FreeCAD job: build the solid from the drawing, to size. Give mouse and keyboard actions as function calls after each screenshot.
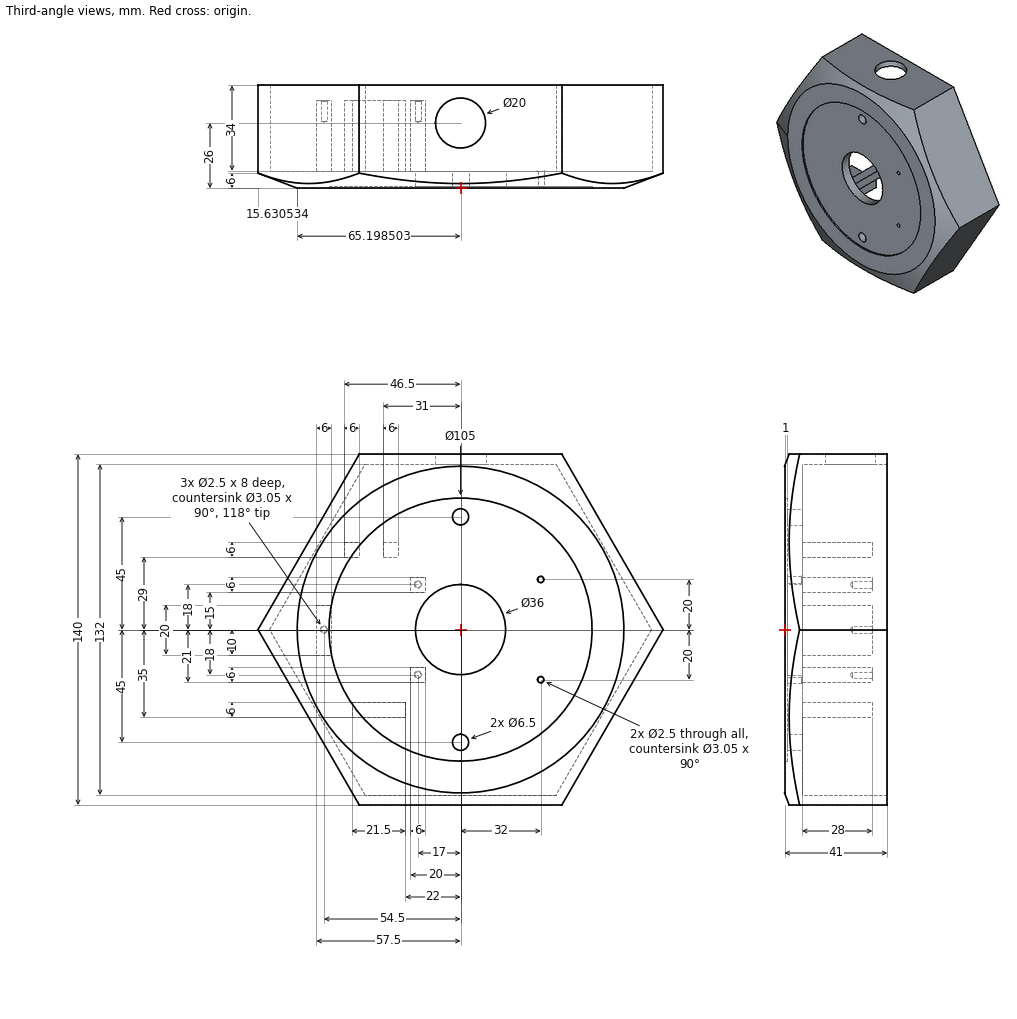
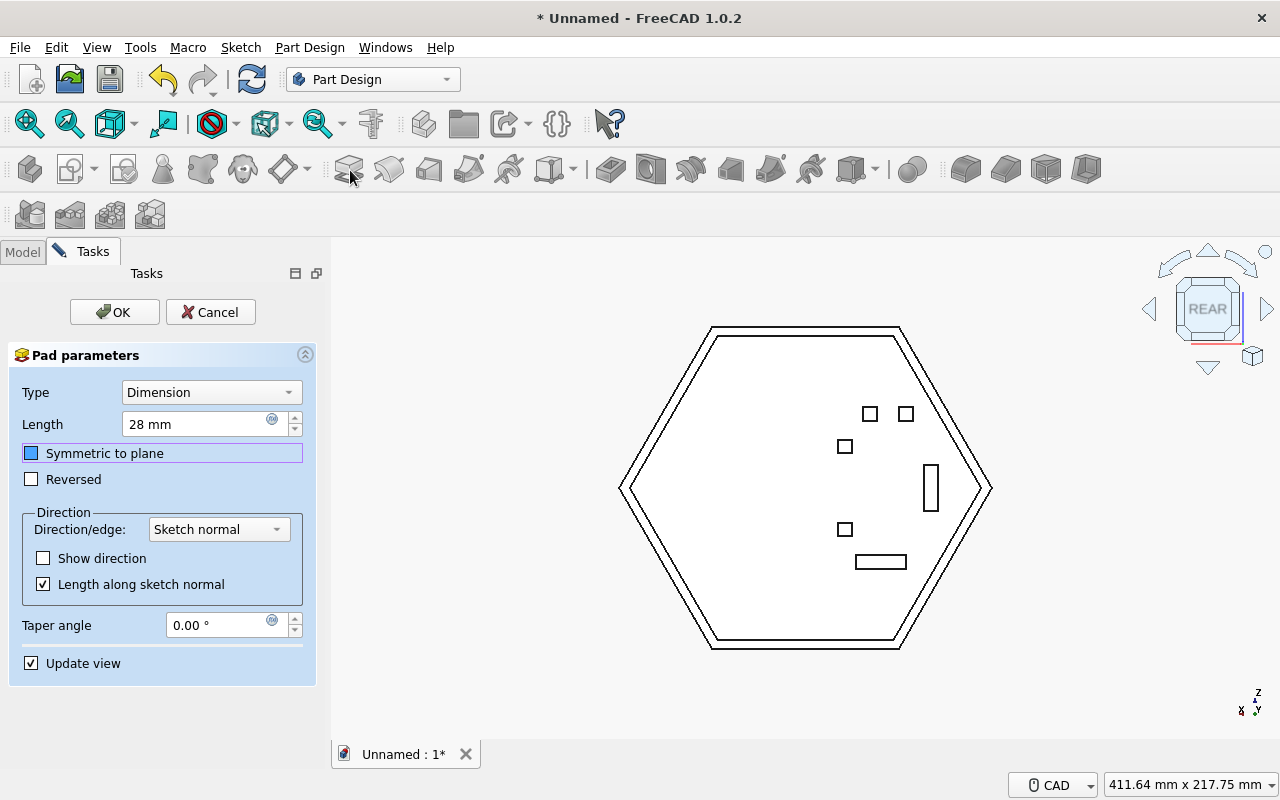
click(115, 312)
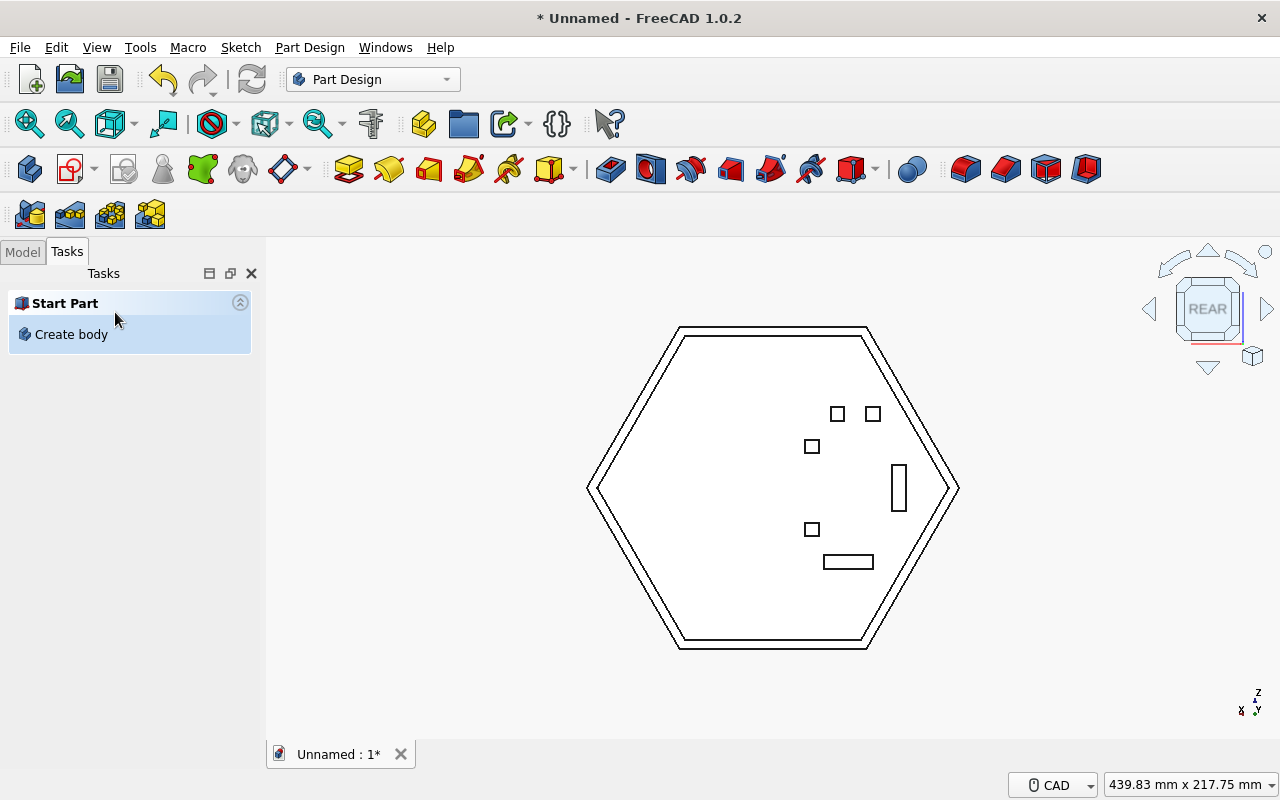
click(723, 487)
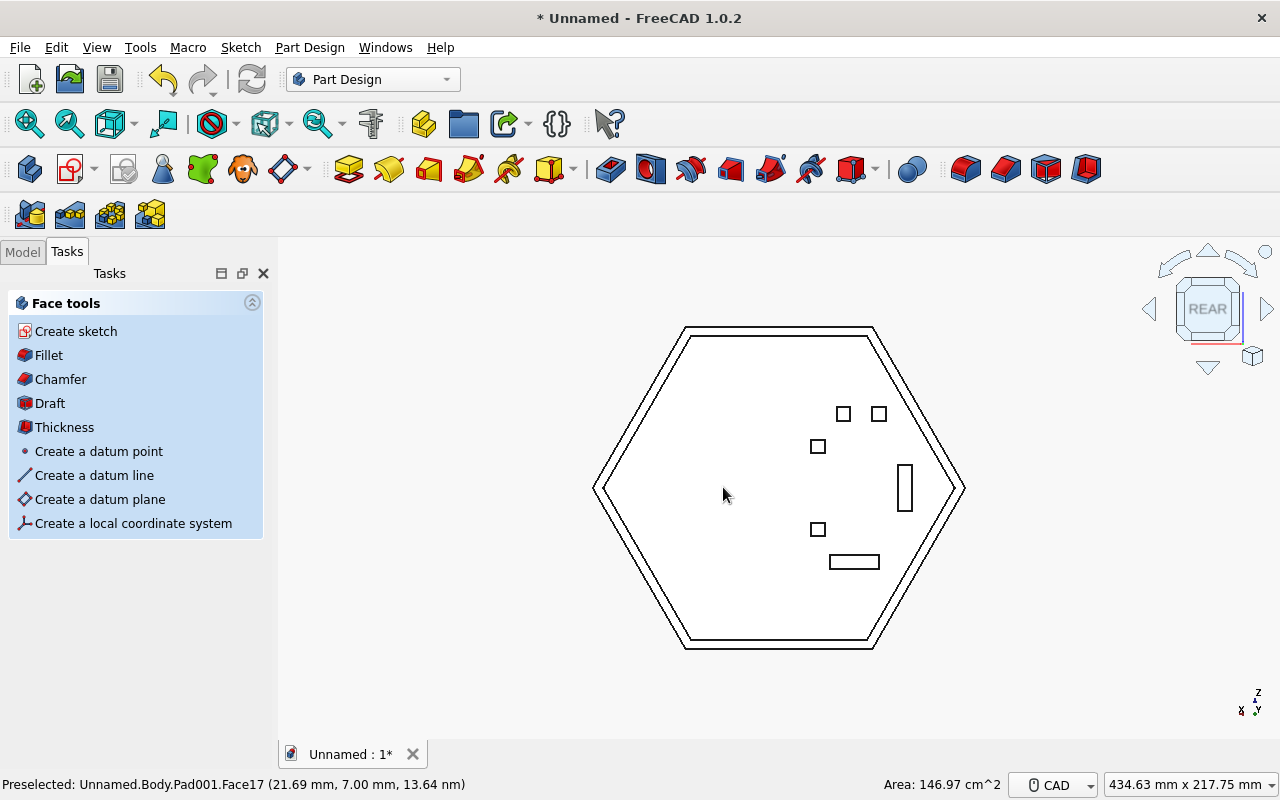
click(70, 170)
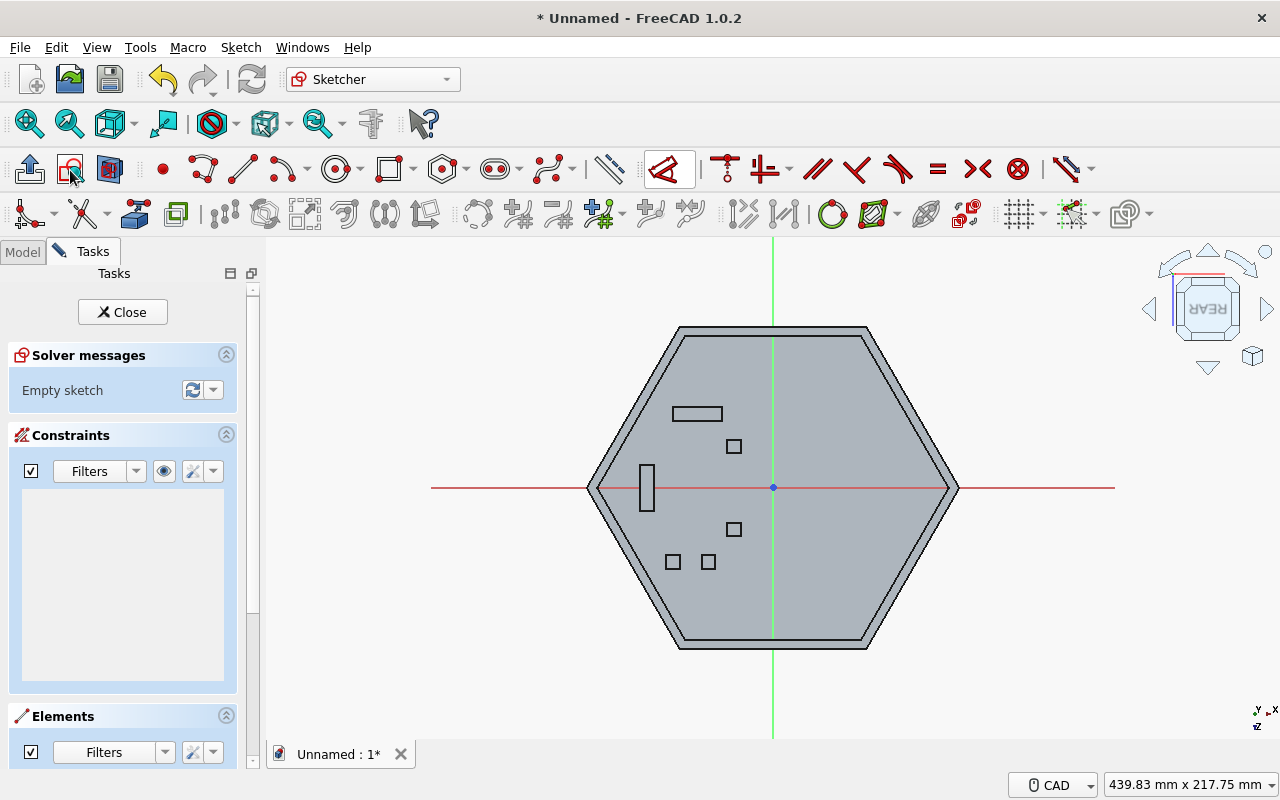
scroll(795, 488, up, 7)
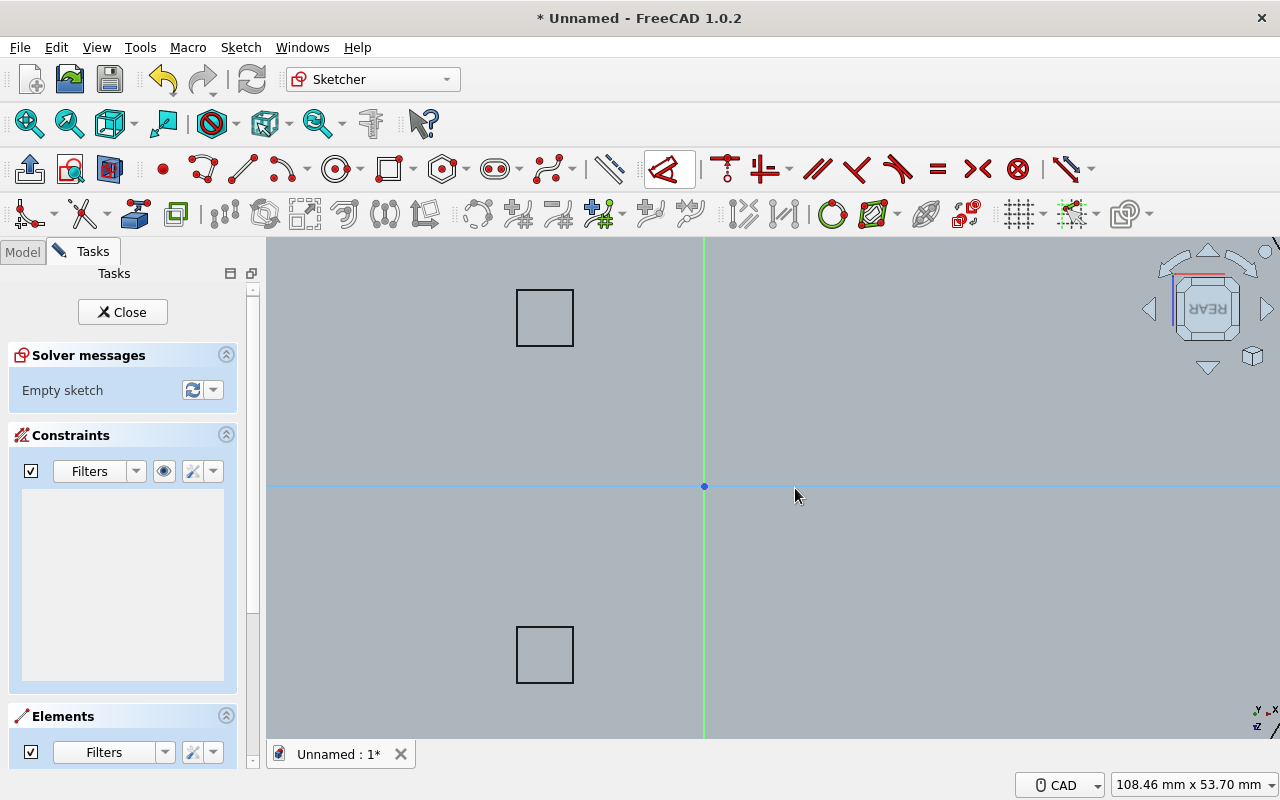
key(g)
key(c)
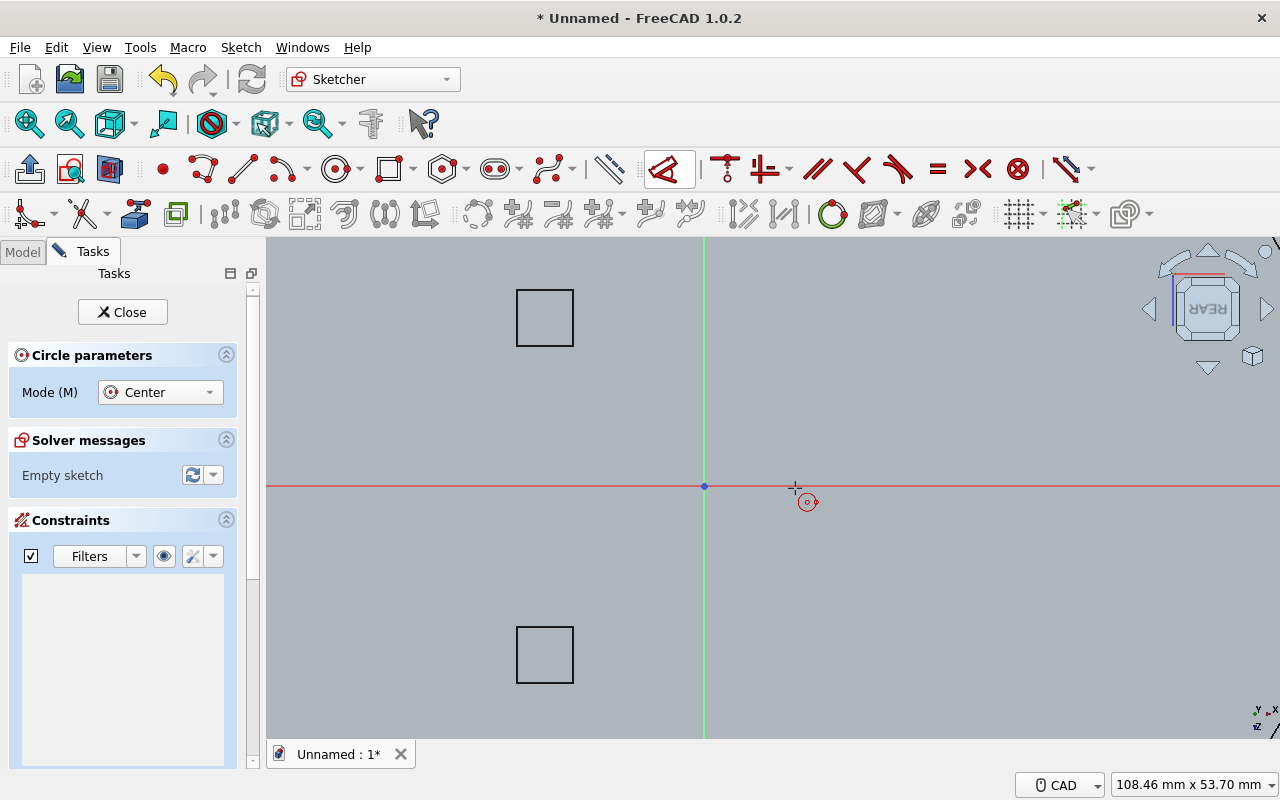
click(704, 486)
move(823, 367)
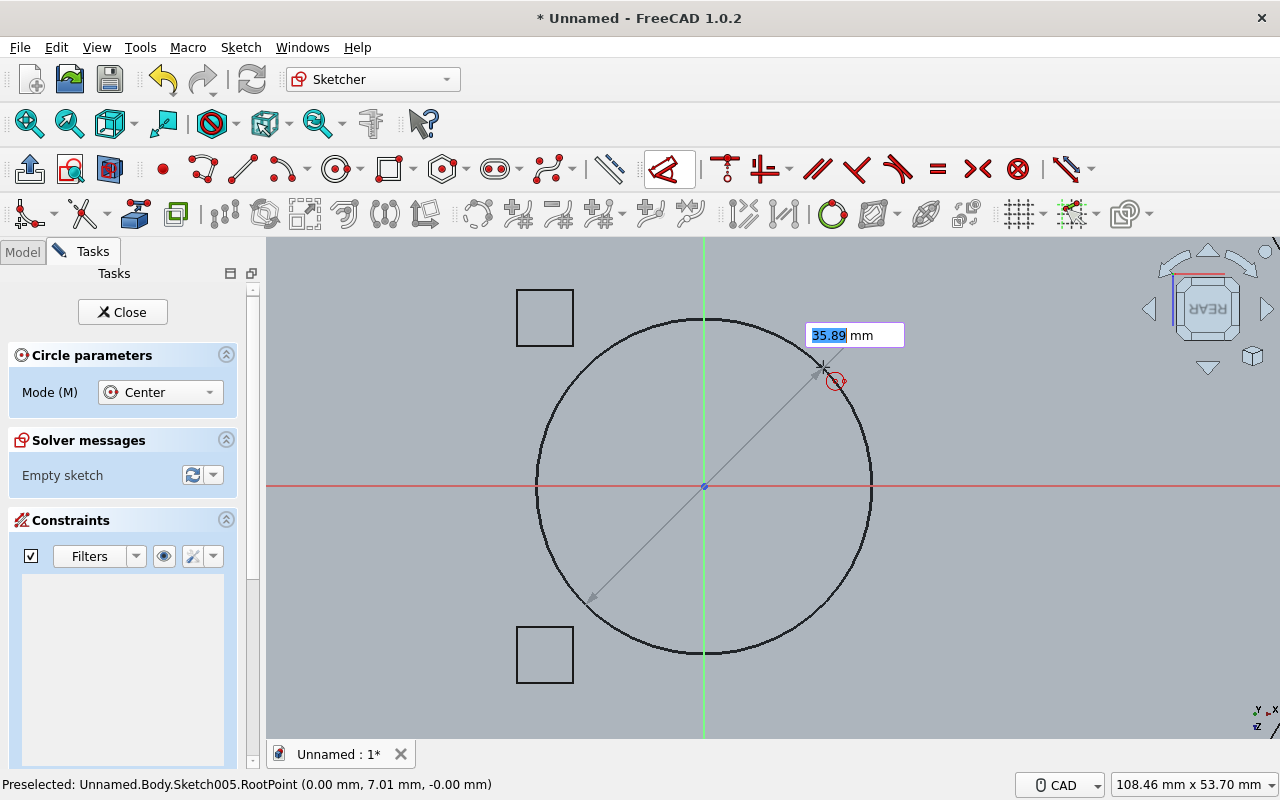
text(36)
key(Return)
key(Escape)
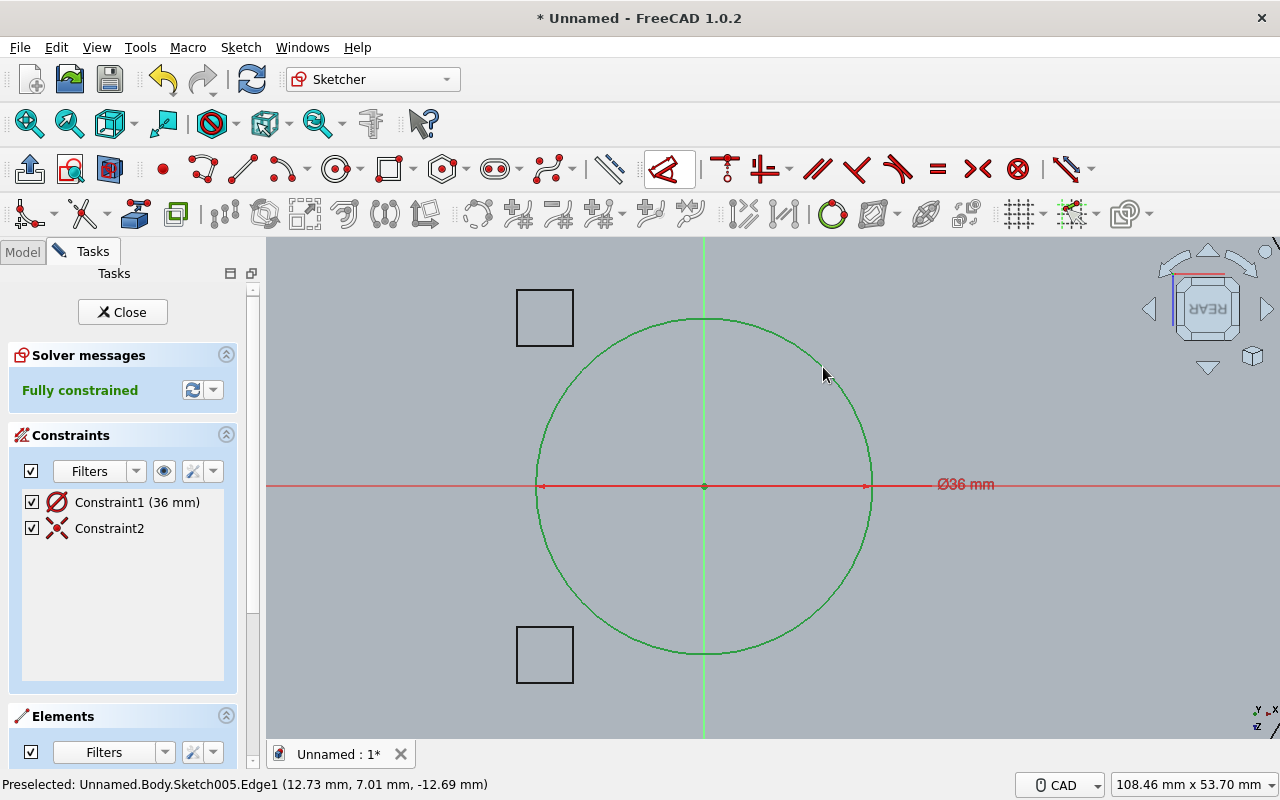
click(123, 312)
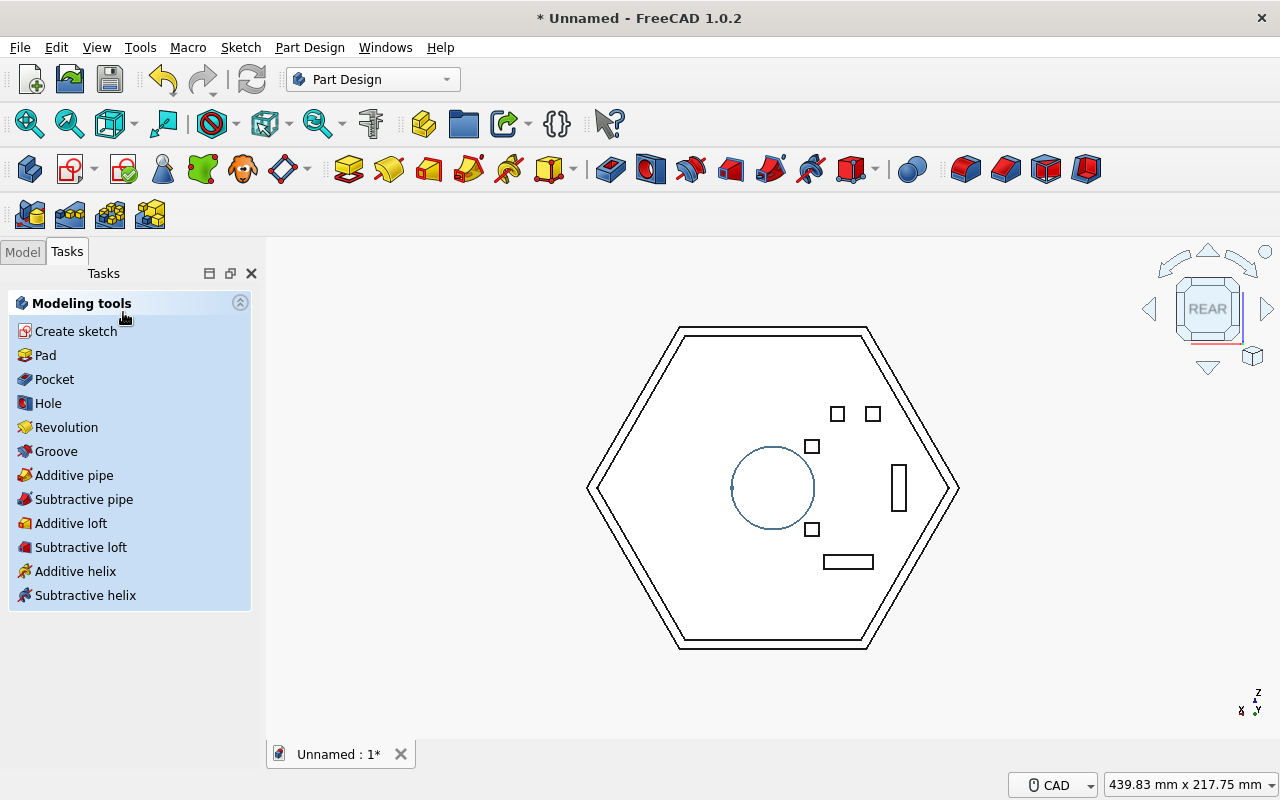
click(612, 170)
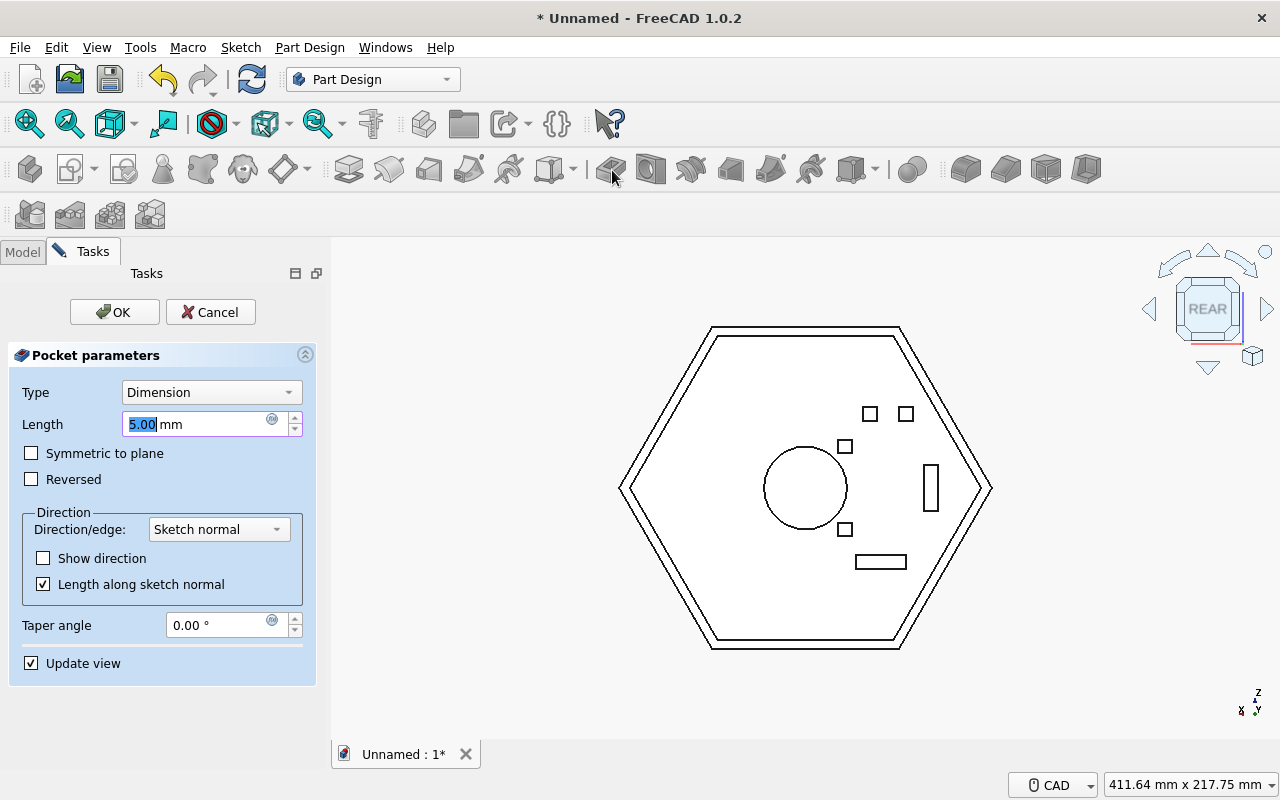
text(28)
key(Tab)